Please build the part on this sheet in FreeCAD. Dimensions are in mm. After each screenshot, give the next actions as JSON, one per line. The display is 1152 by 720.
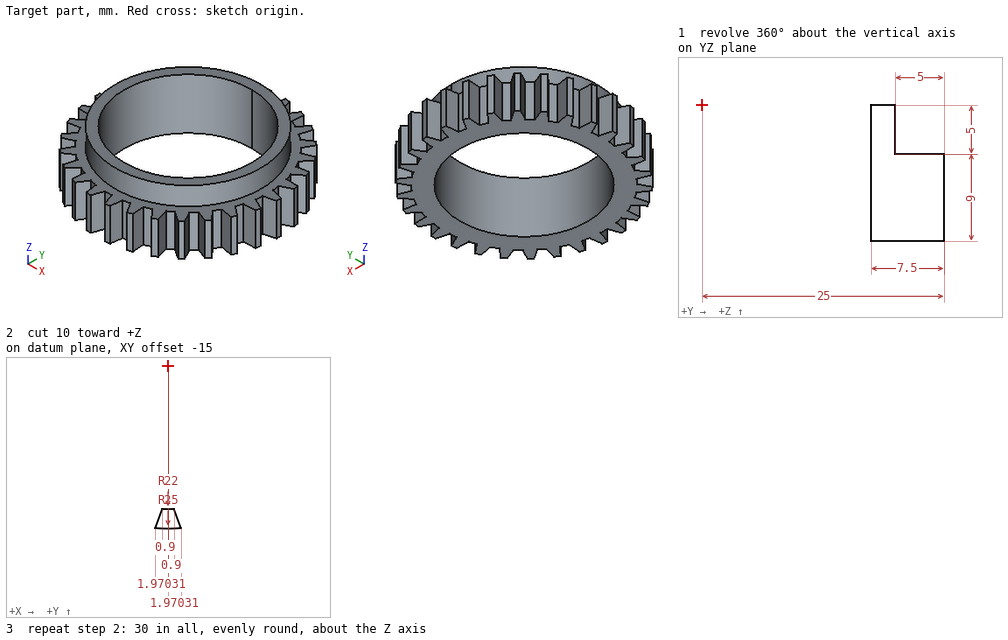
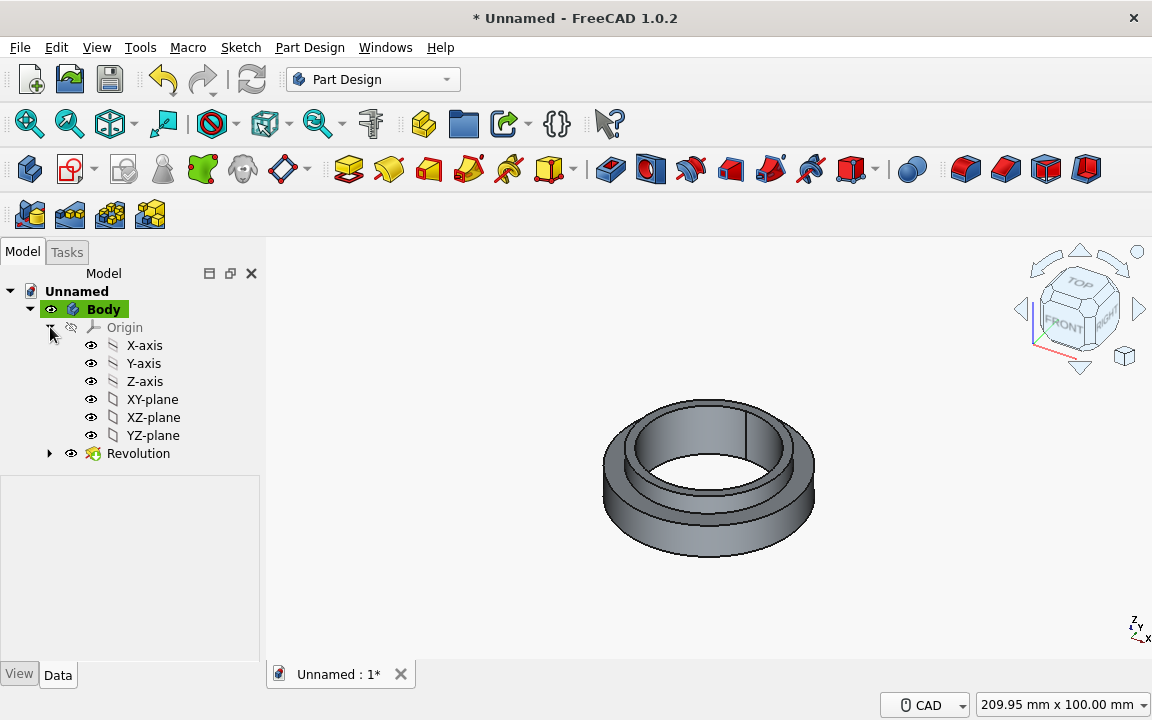
{"action": "left_click", "coordinate": [136, 399]}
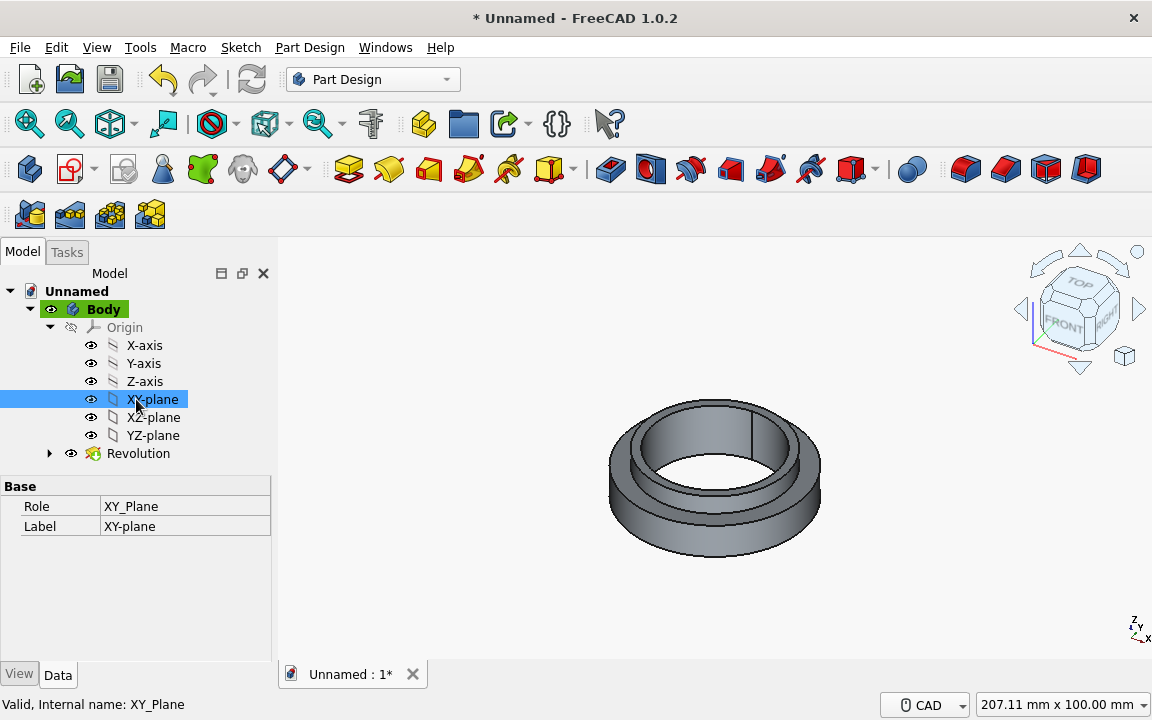
{"action": "left_click", "coordinate": [284, 170]}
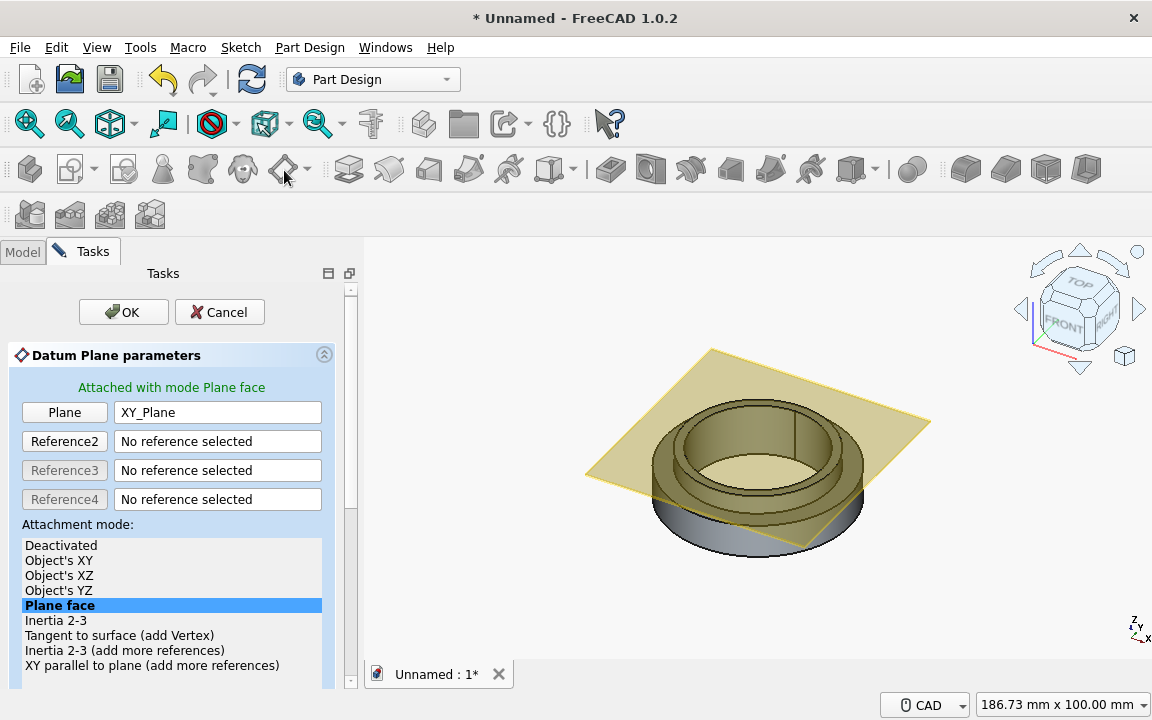
{"action": "scroll", "coordinate": [351, 486], "scroll_direction": "down", "scroll_amount": 4}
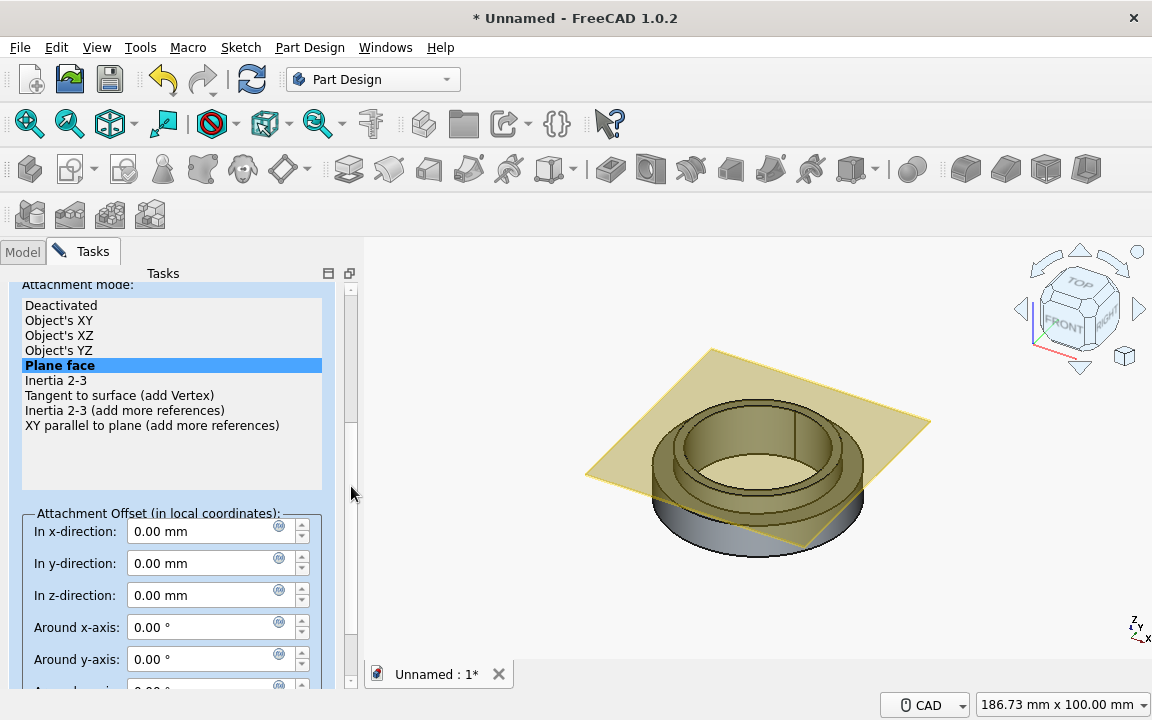
{"action": "triple_click", "coordinate": [210, 595]}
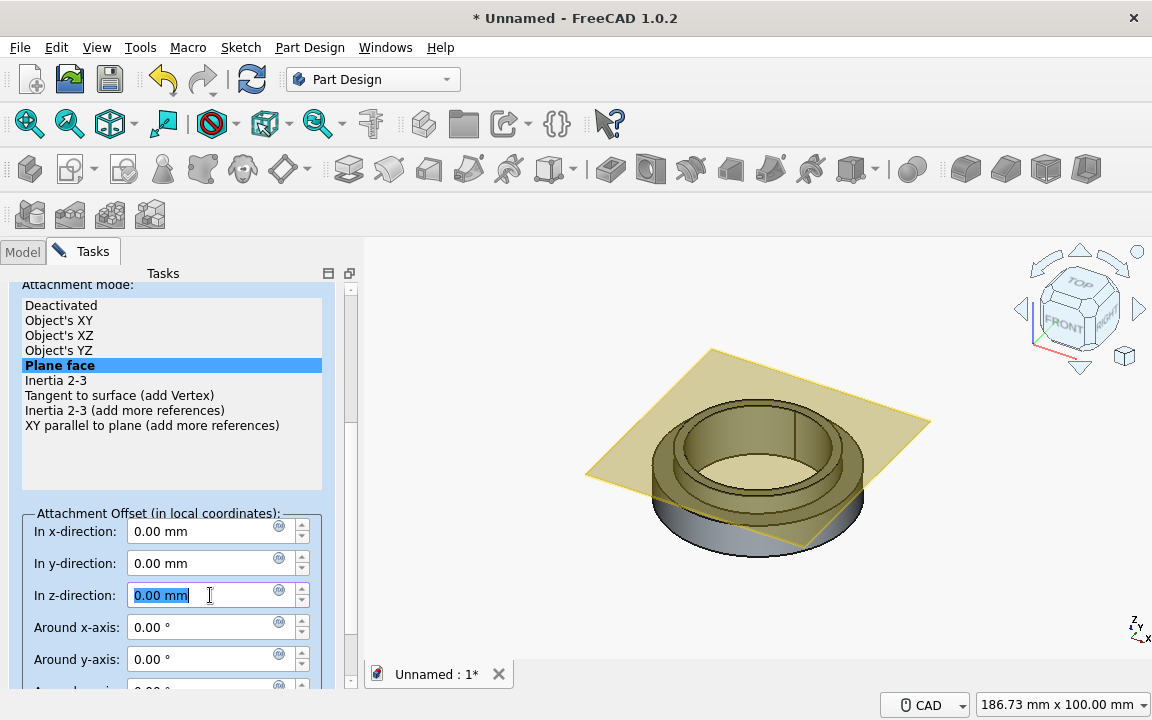
{"action": "type", "text": "-15"}
{"action": "key", "text": "Tab"}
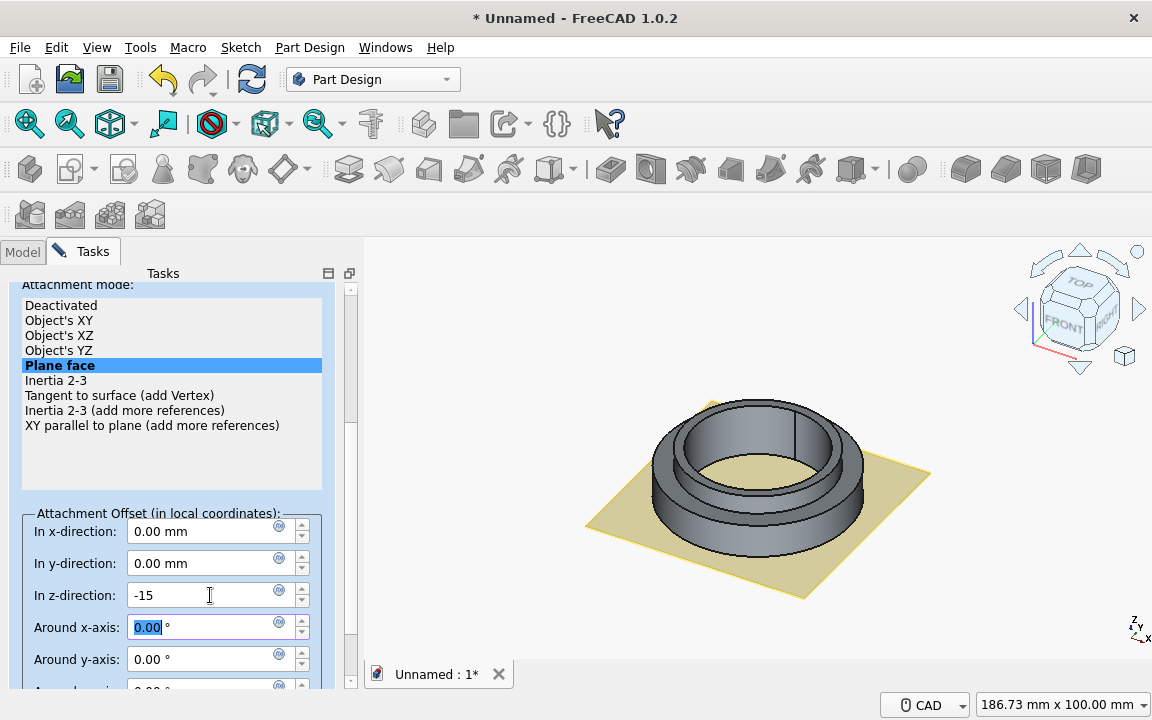
{"action": "scroll", "coordinate": [351, 486], "scroll_direction": "up", "scroll_amount": 5}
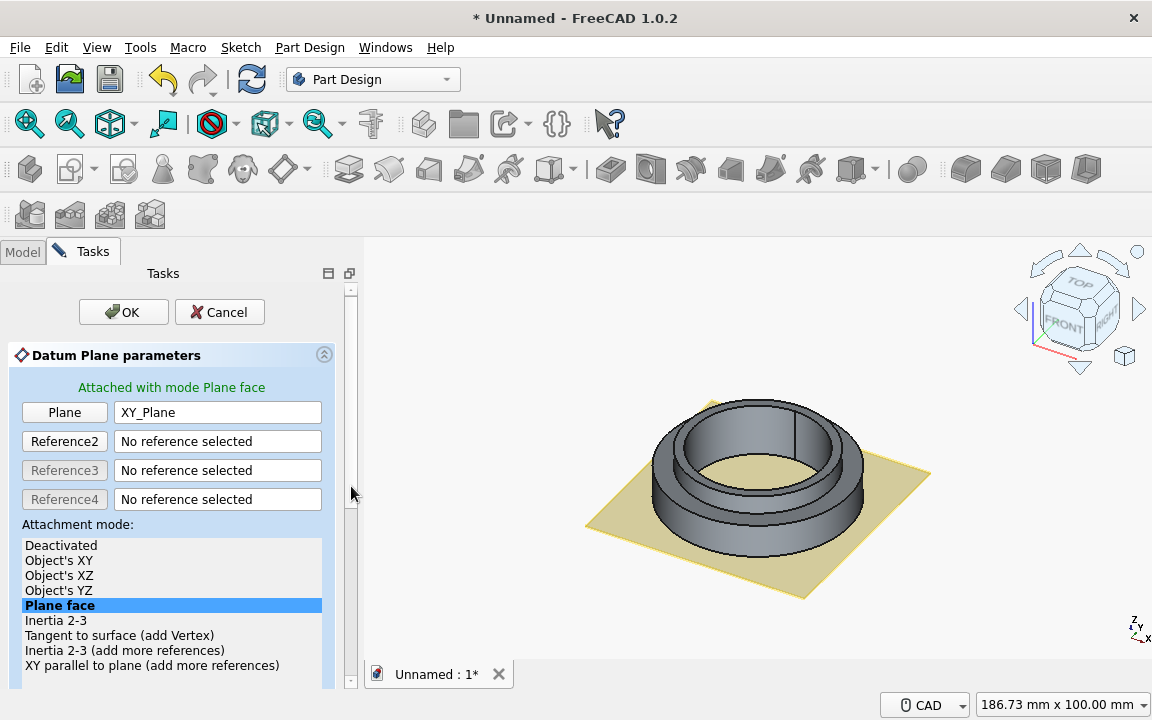
{"action": "left_click", "coordinate": [124, 312]}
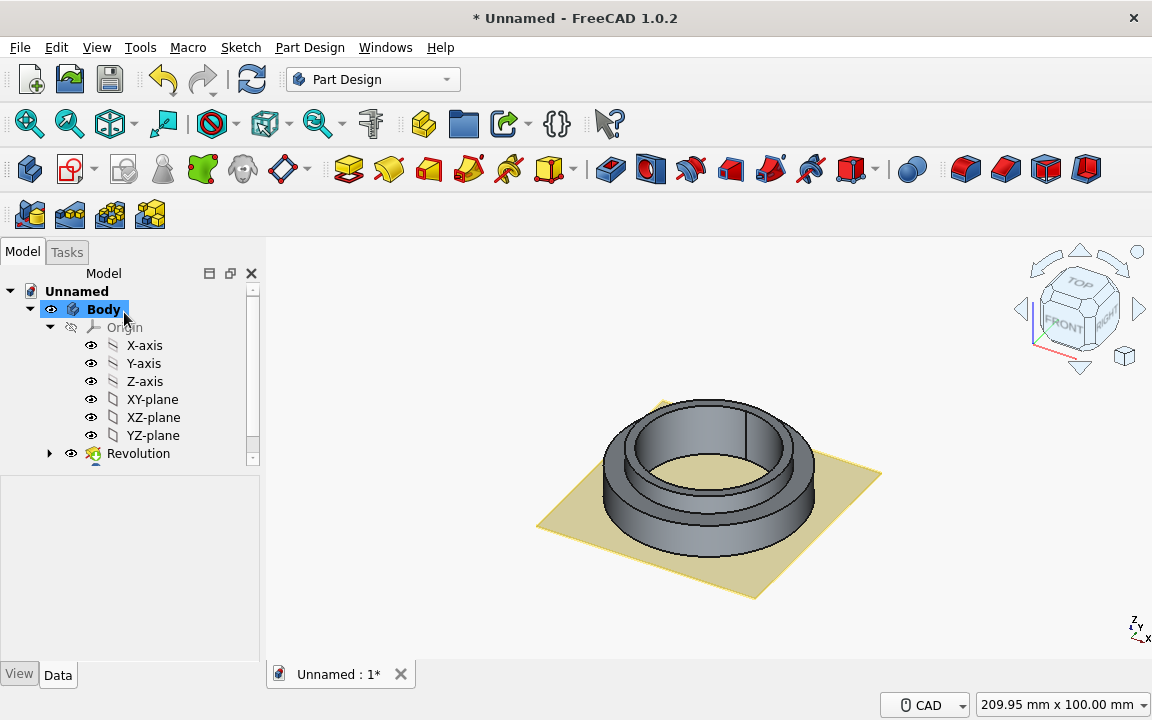
{"action": "scroll", "coordinate": [100, 377], "scroll_direction": "down", "scroll_amount": 3}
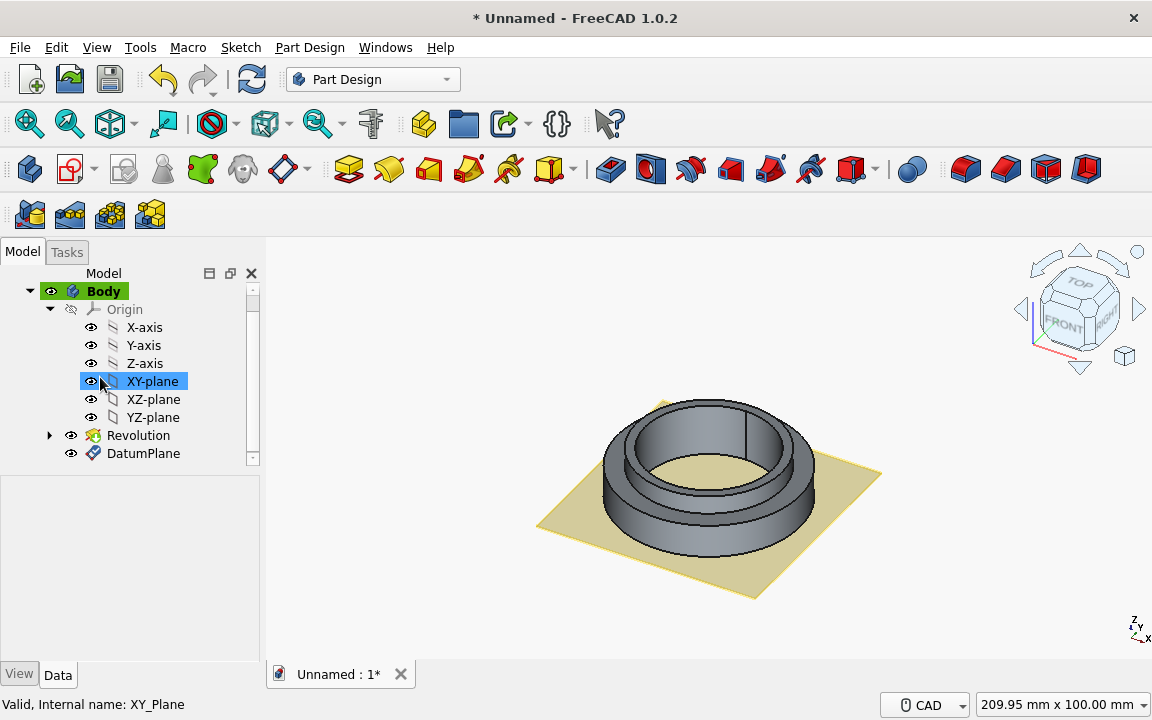
{"action": "left_click", "coordinate": [116, 453]}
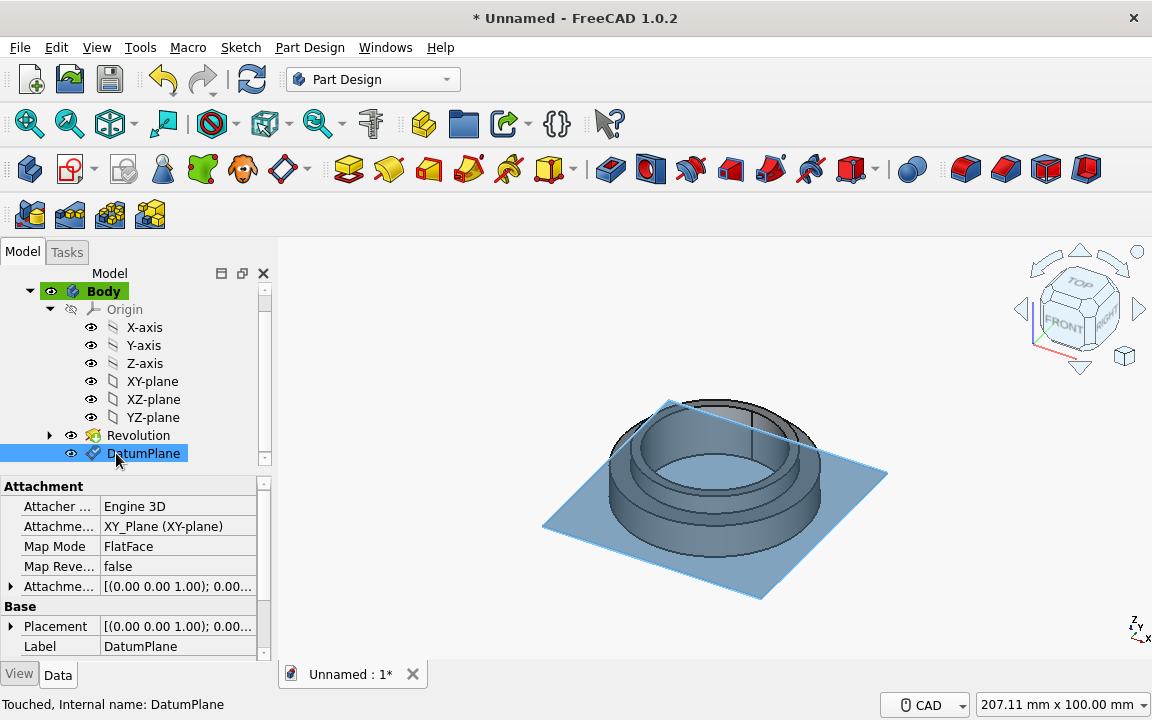
{"action": "left_click", "coordinate": [70, 170]}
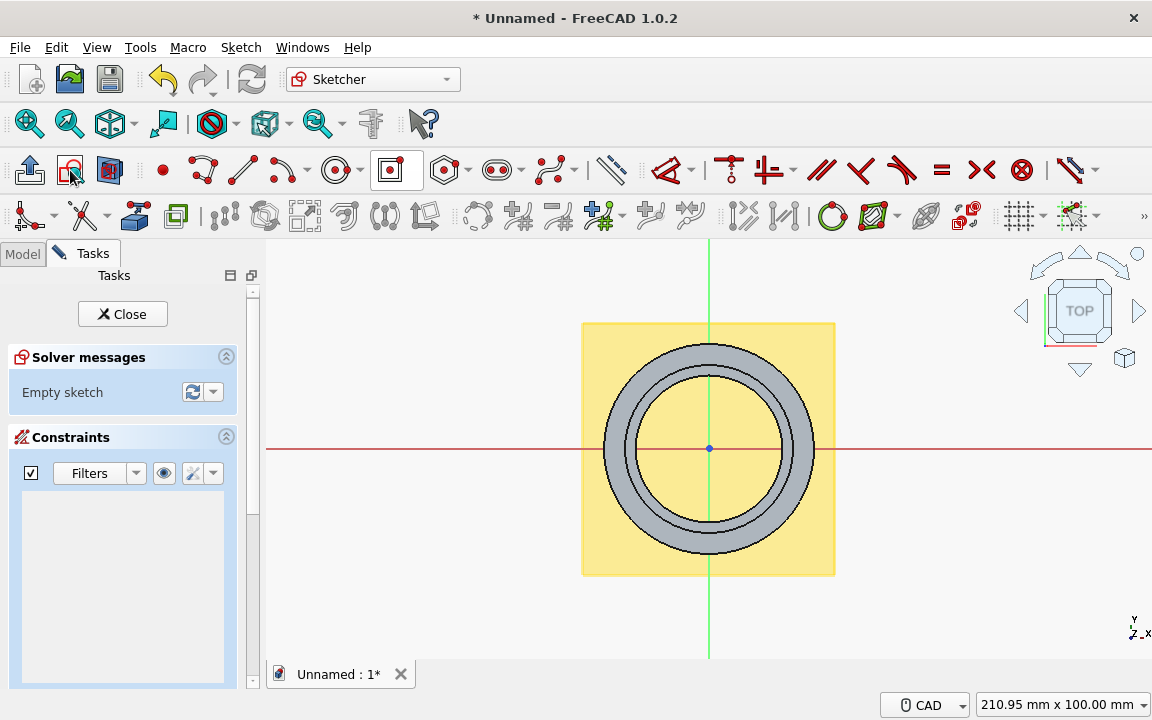
{"action": "left_click", "coordinate": [110, 170]}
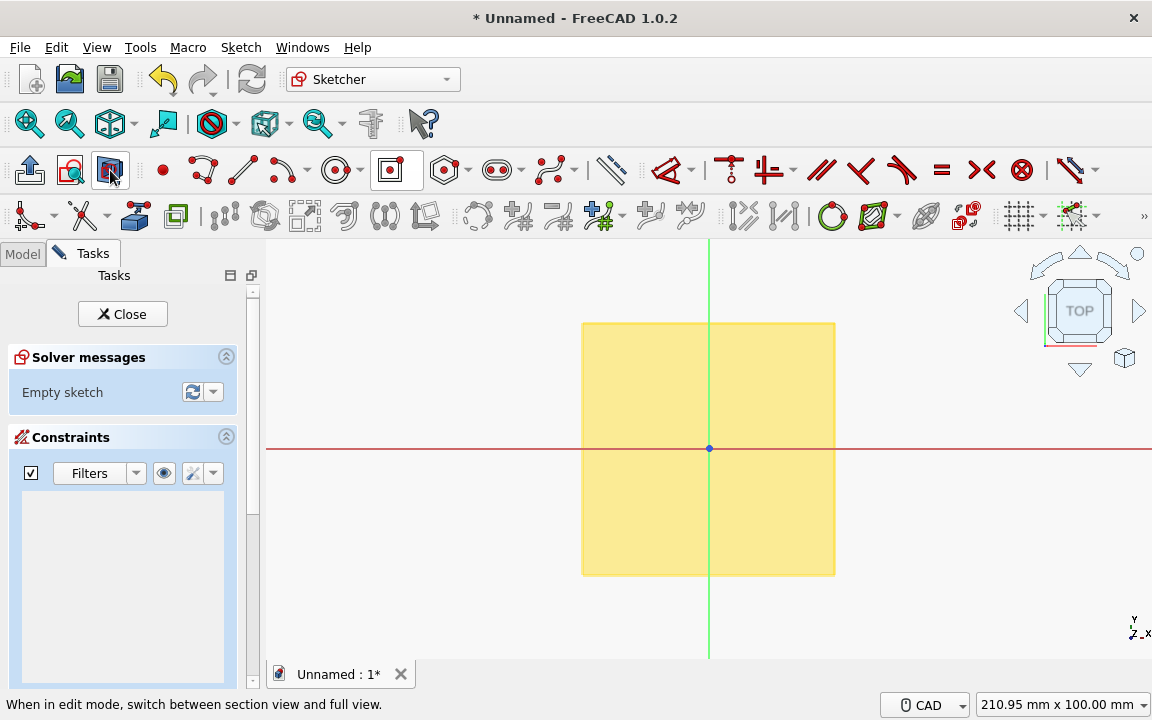
{"action": "scroll", "coordinate": [713, 553], "scroll_direction": "up", "scroll_amount": 15}